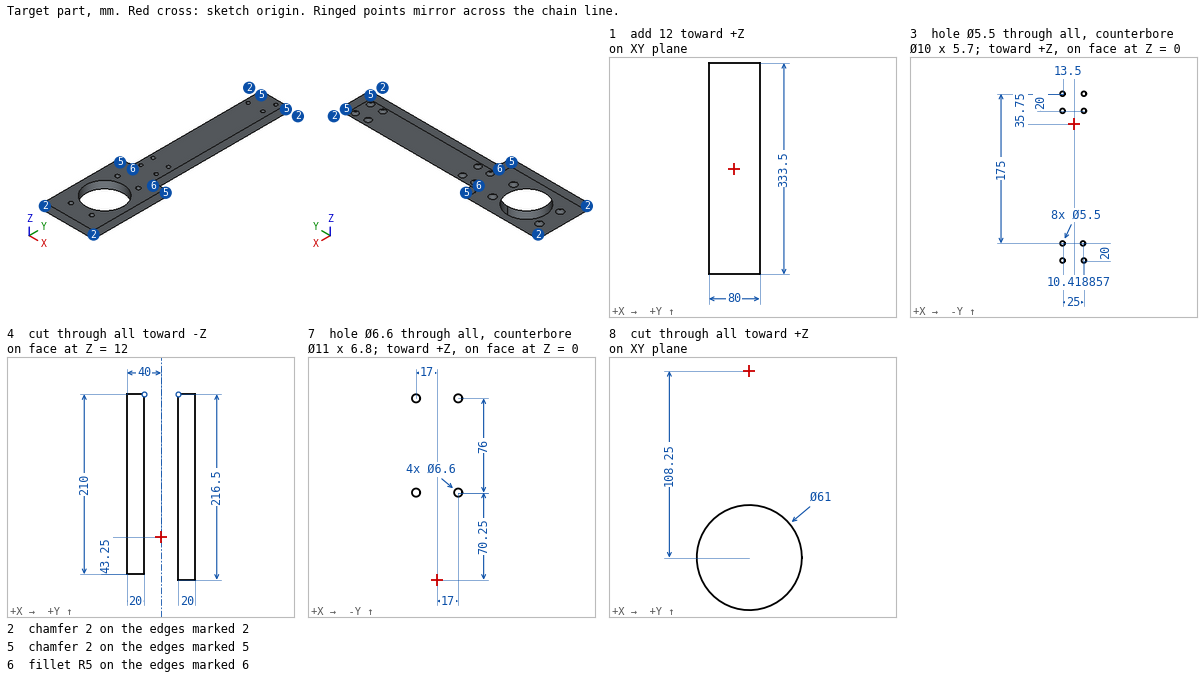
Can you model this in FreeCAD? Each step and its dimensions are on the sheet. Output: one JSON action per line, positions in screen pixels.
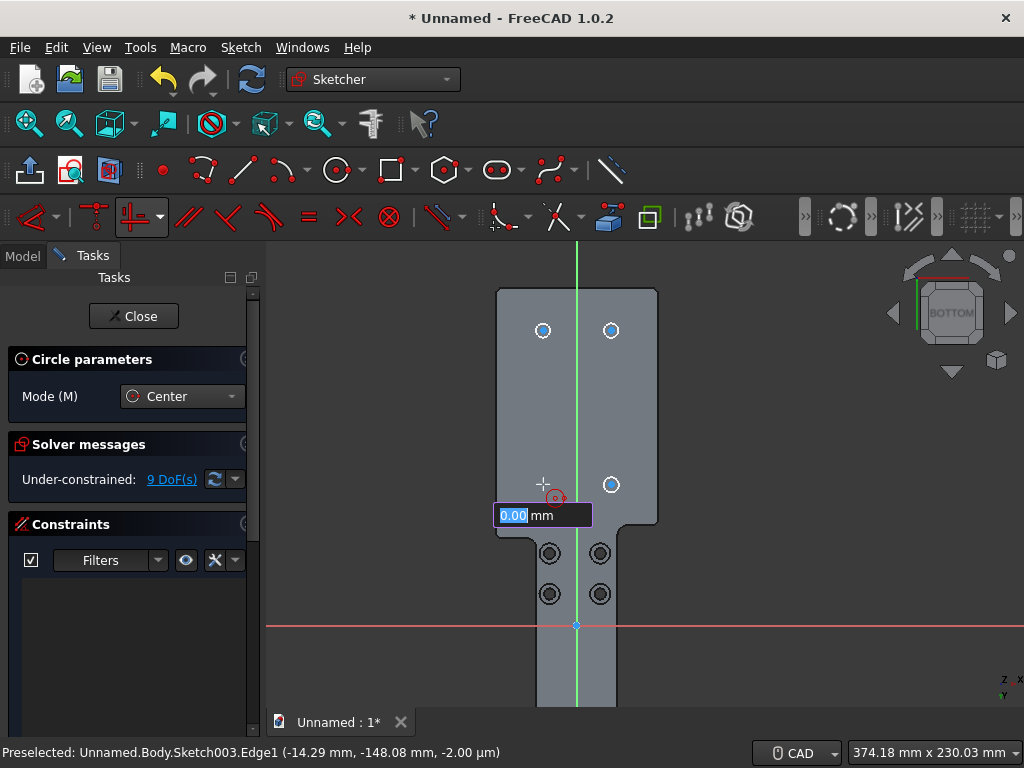
{"action": "scroll", "coordinate": [547, 479], "scroll_direction": "up", "scroll_amount": 5}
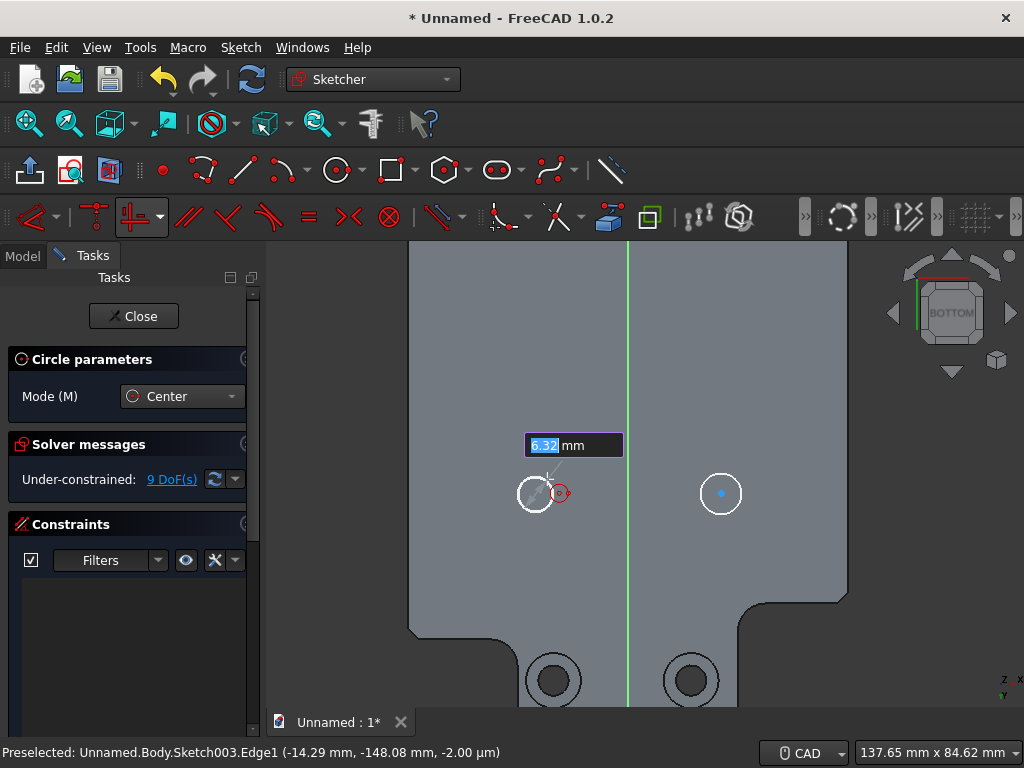
{"action": "left_click", "coordinate": [547, 478]}
{"action": "key", "text": "Escape"}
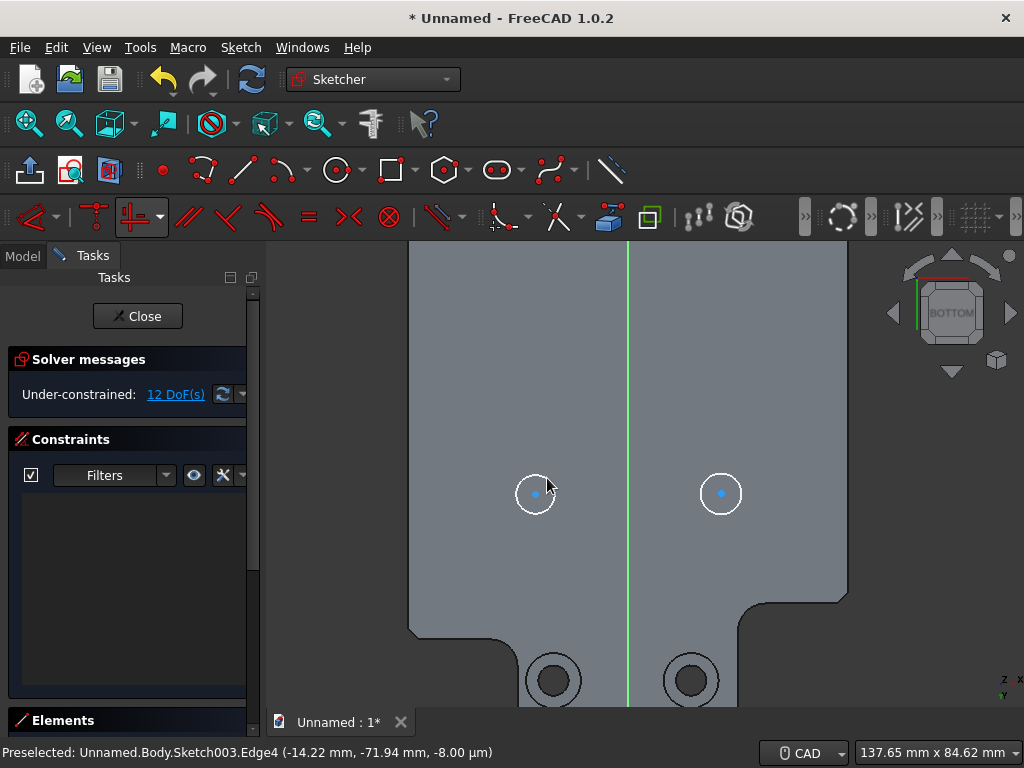
{"action": "left_click", "coordinate": [735, 479]}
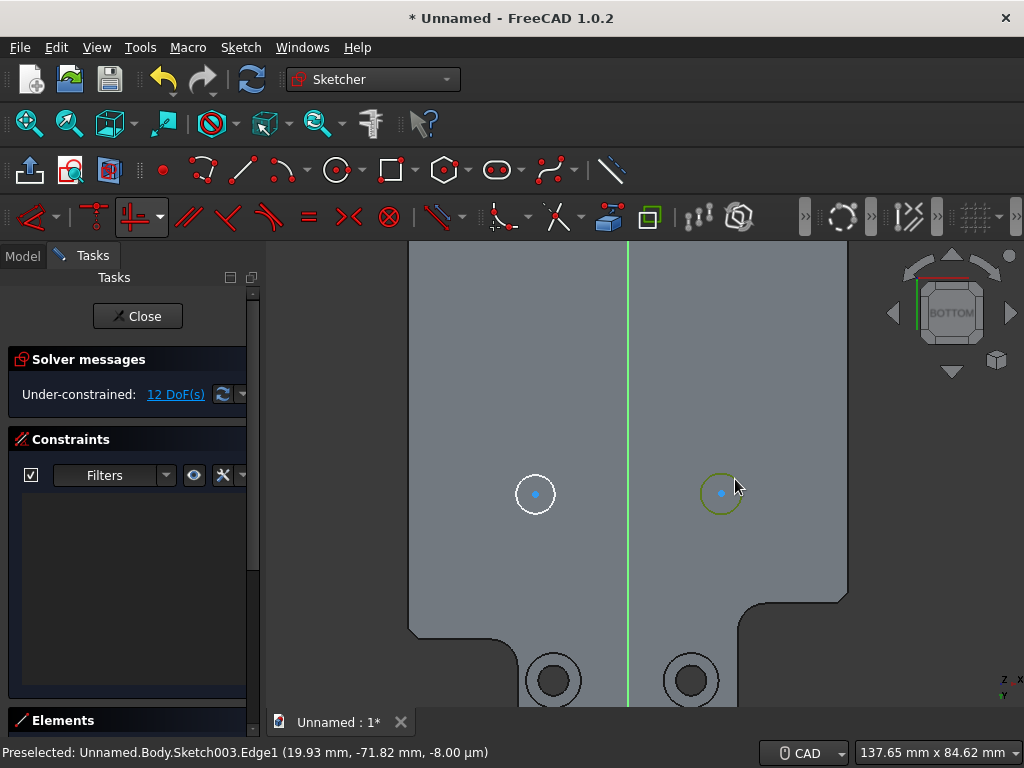
{"action": "scroll", "coordinate": [547, 479], "scroll_direction": "down", "scroll_amount": 5}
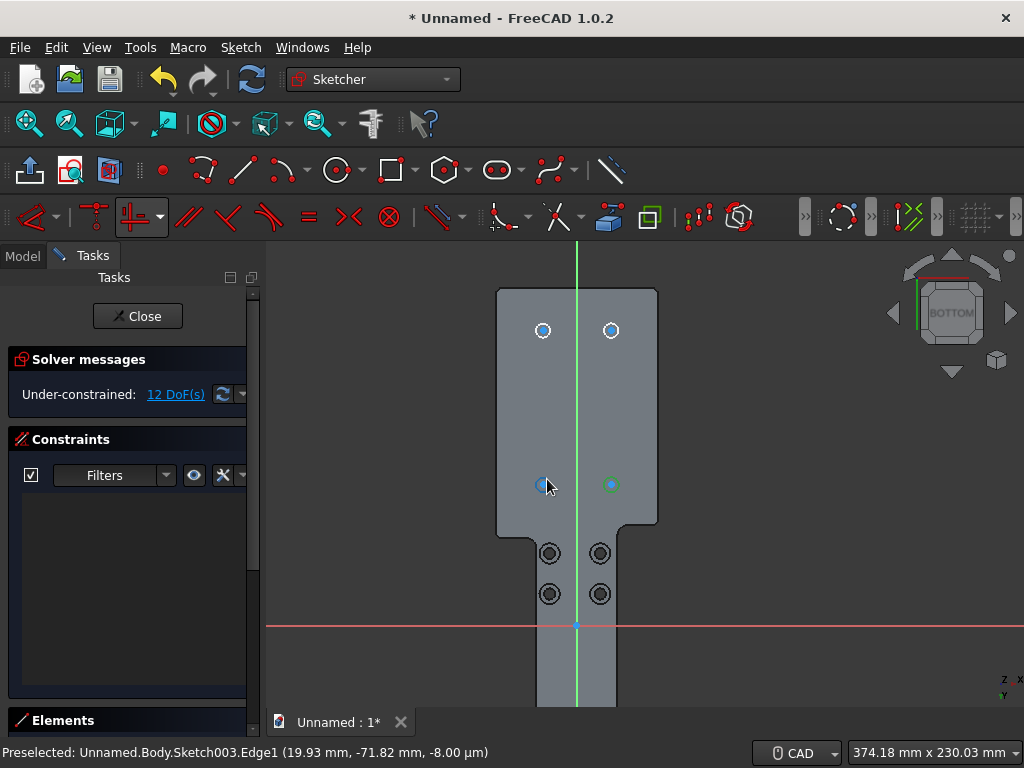
{"action": "scroll", "coordinate": [616, 326], "scroll_direction": "up", "scroll_amount": 4}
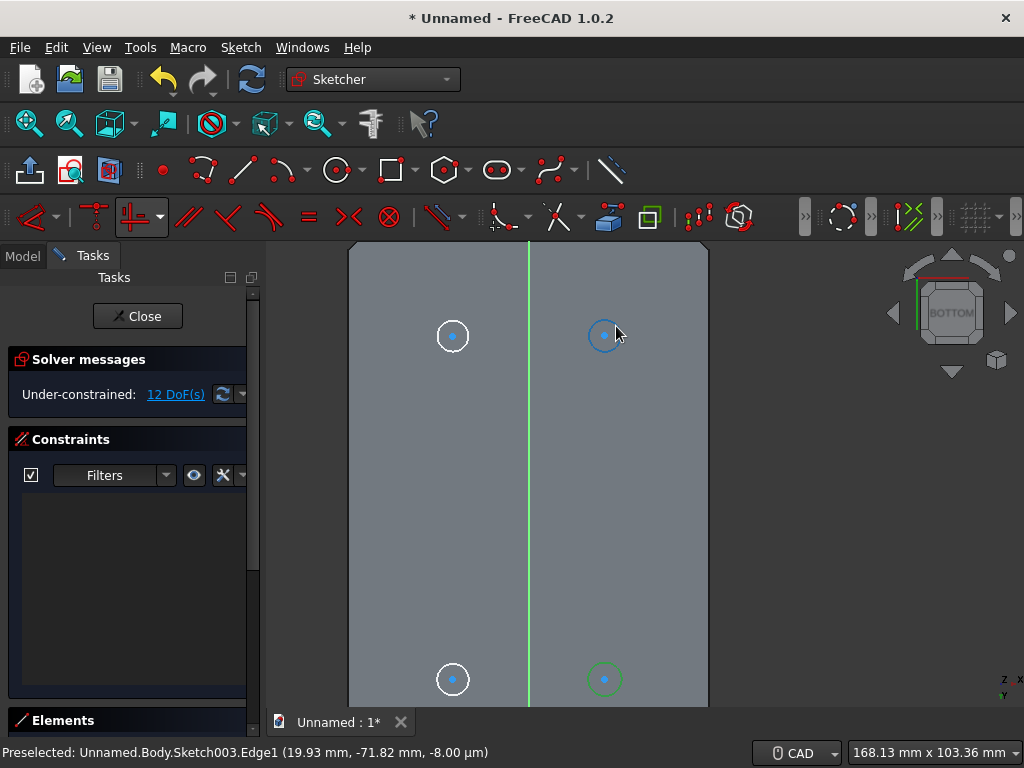
{"action": "left_click", "coordinate": [616, 325]}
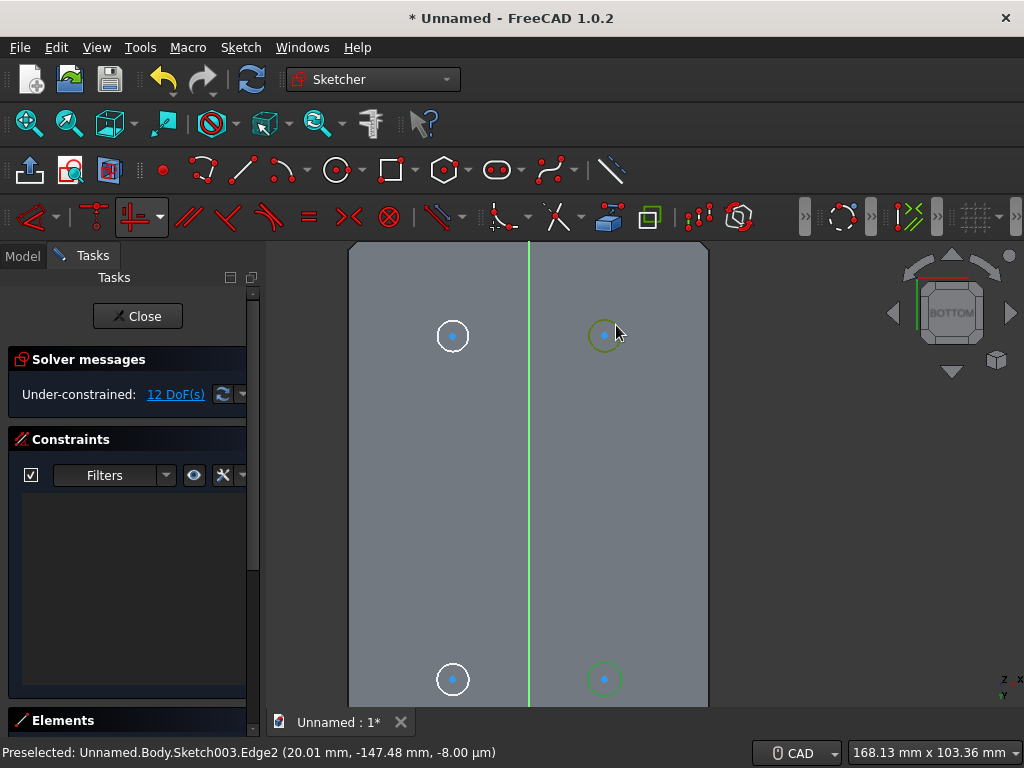
{"action": "left_click", "coordinate": [464, 325]}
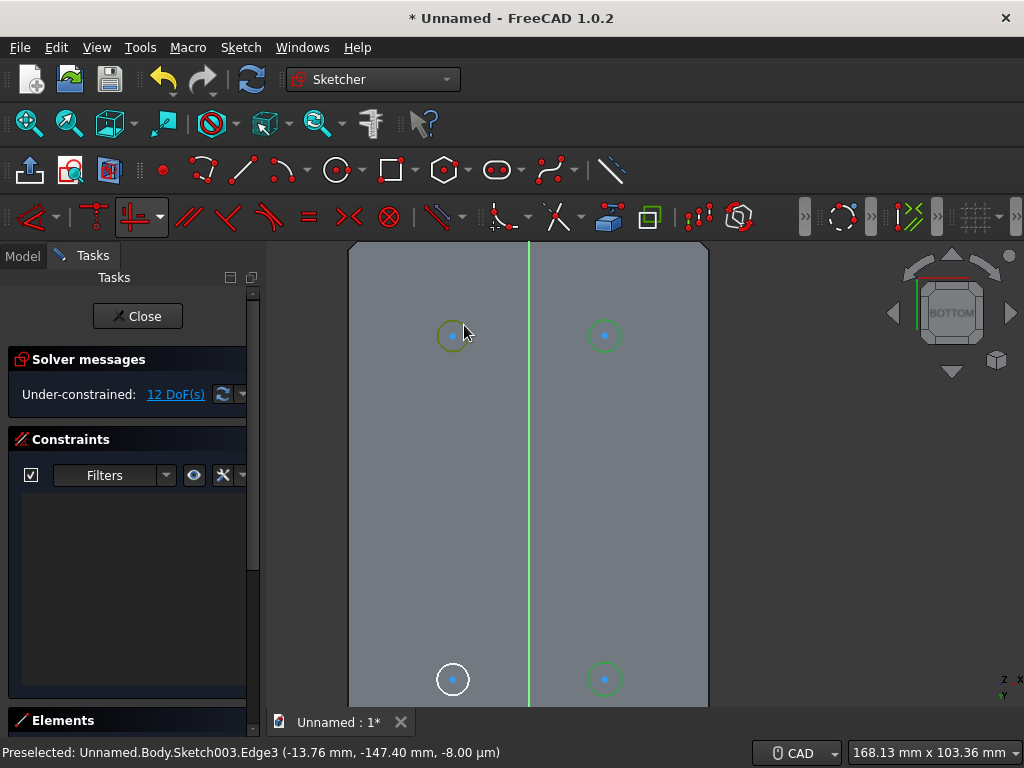
{"action": "left_click", "coordinate": [464, 668]}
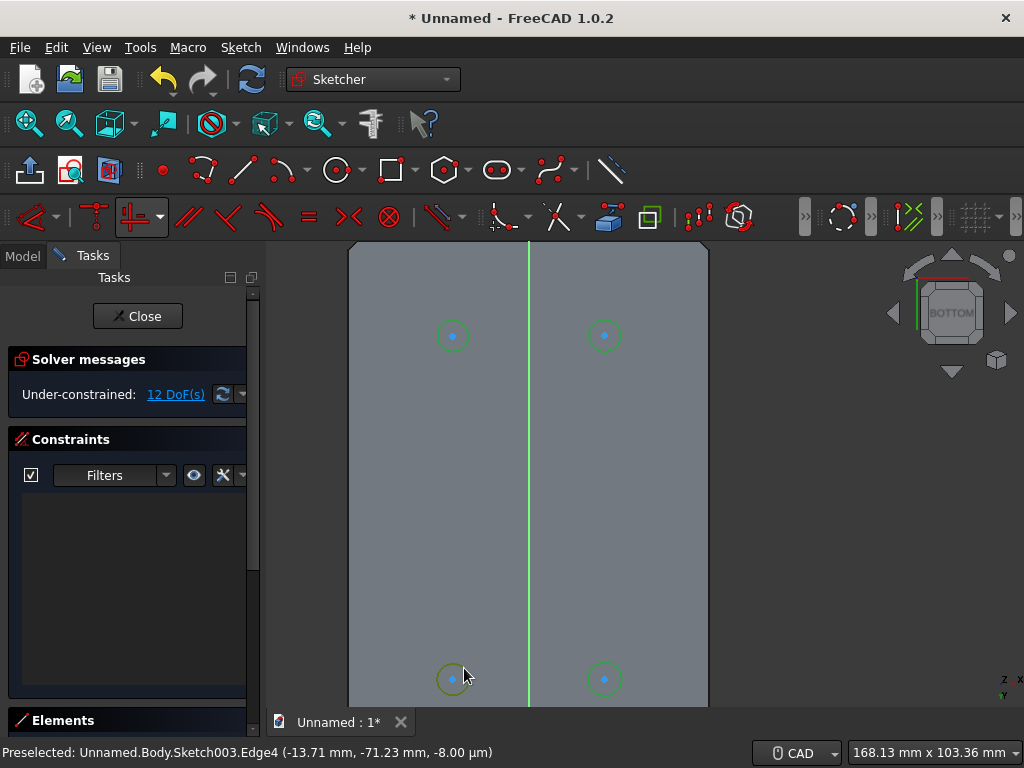
{"action": "key", "text": "e"}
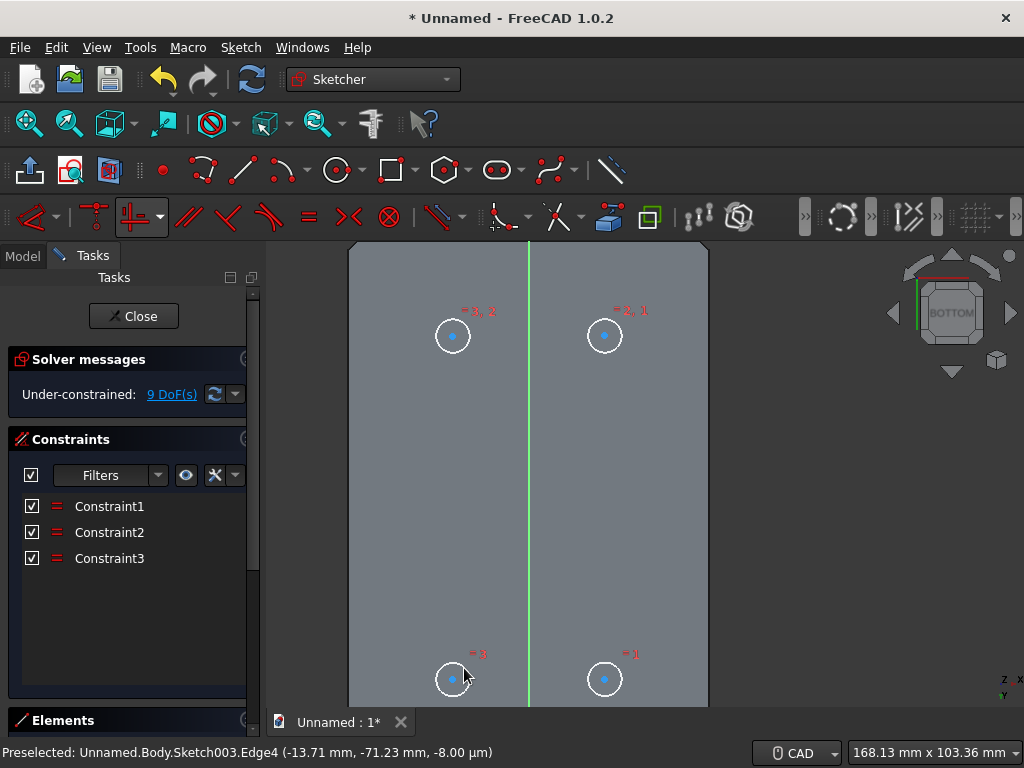
{"action": "scroll", "coordinate": [616, 325], "scroll_direction": "down", "scroll_amount": 4}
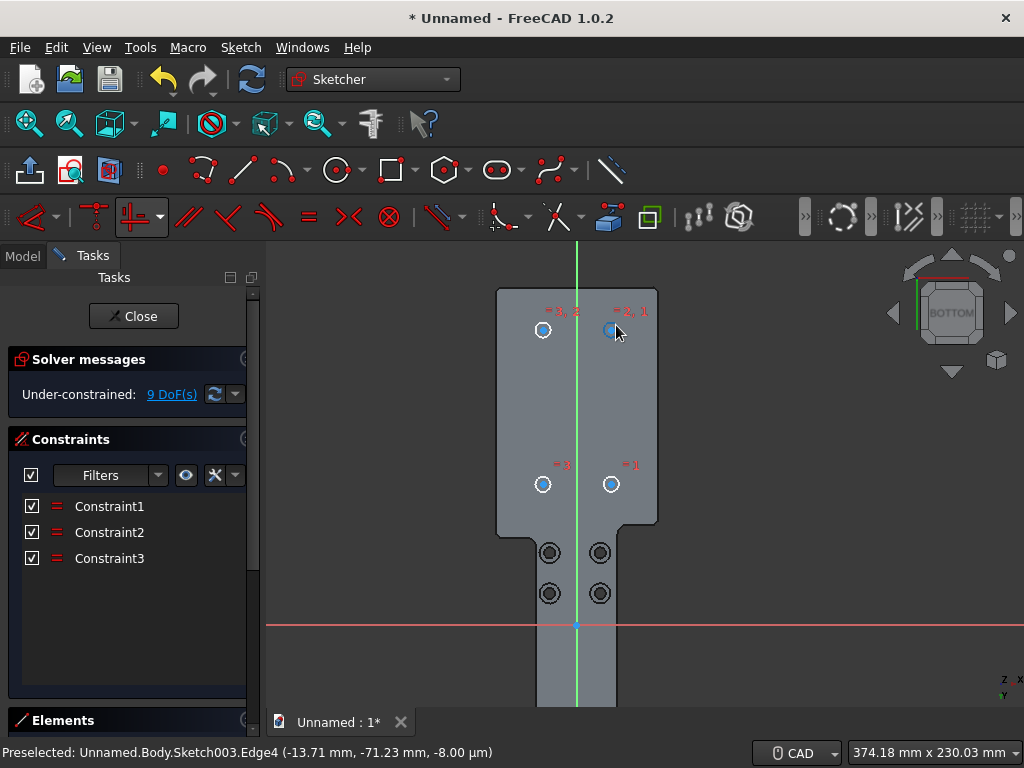
{"action": "left_click", "coordinate": [611, 484]}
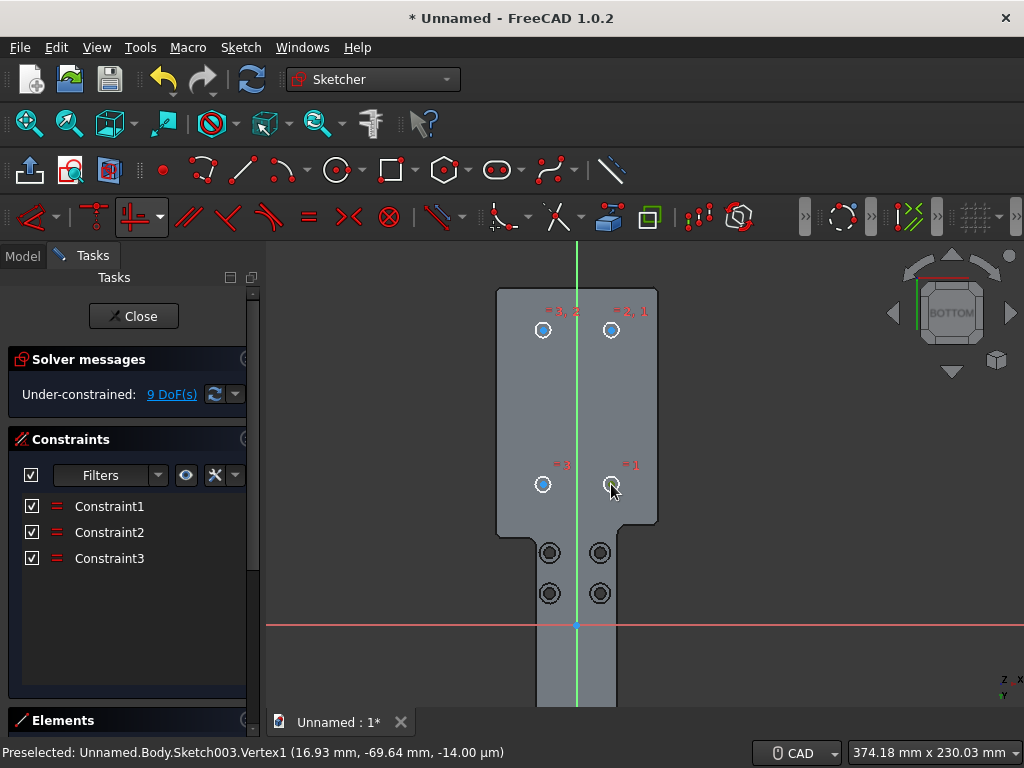
{"action": "left_click", "coordinate": [611, 330]}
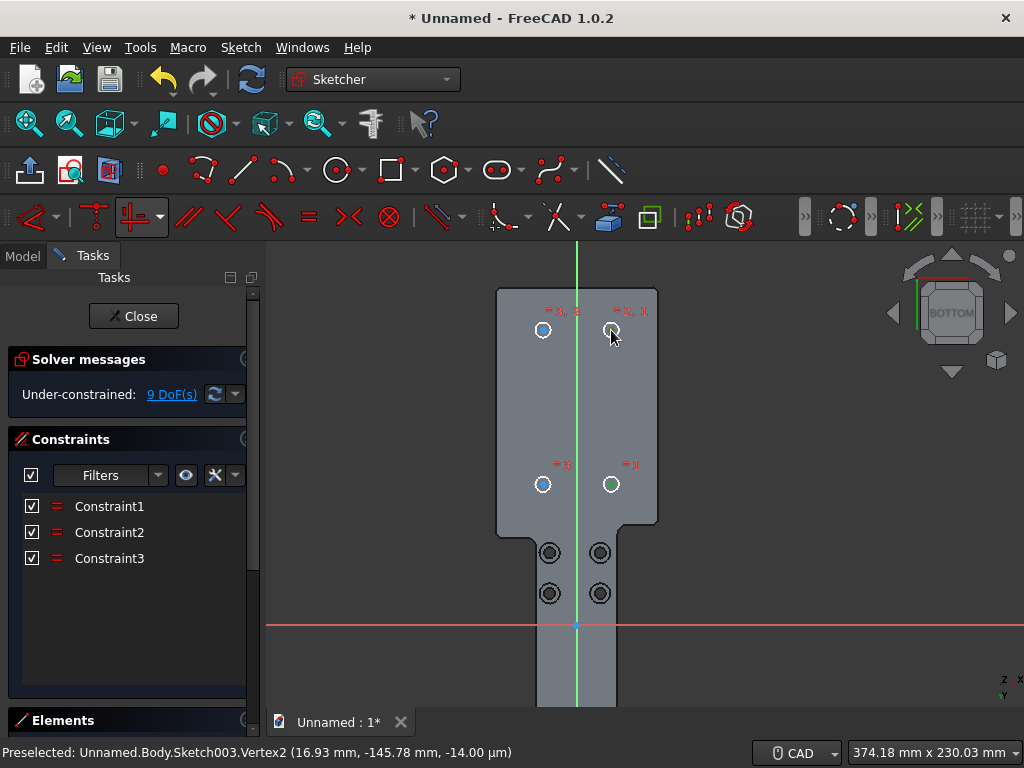
{"action": "key", "text": "v"}